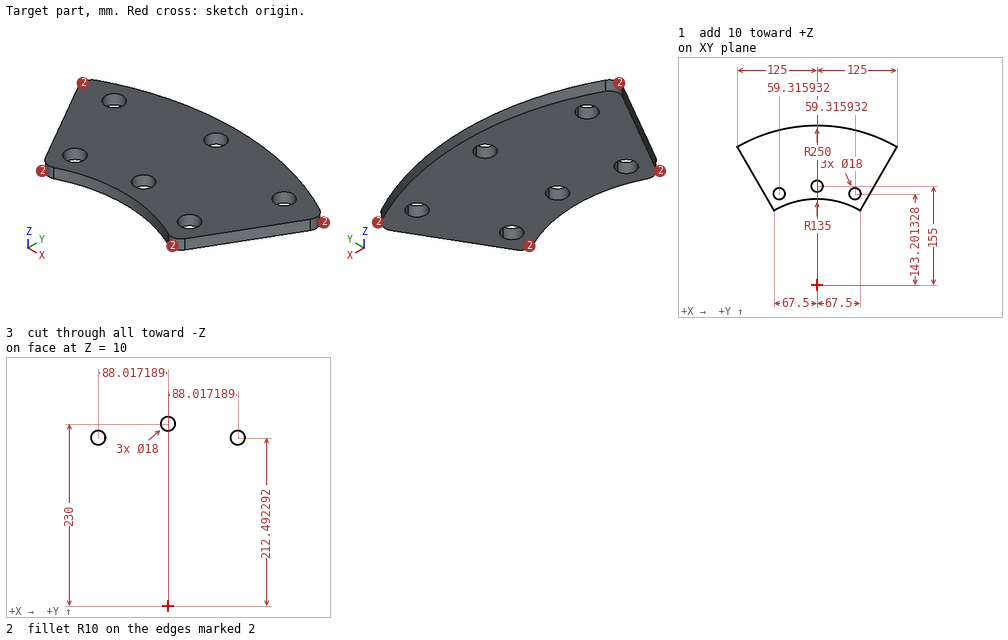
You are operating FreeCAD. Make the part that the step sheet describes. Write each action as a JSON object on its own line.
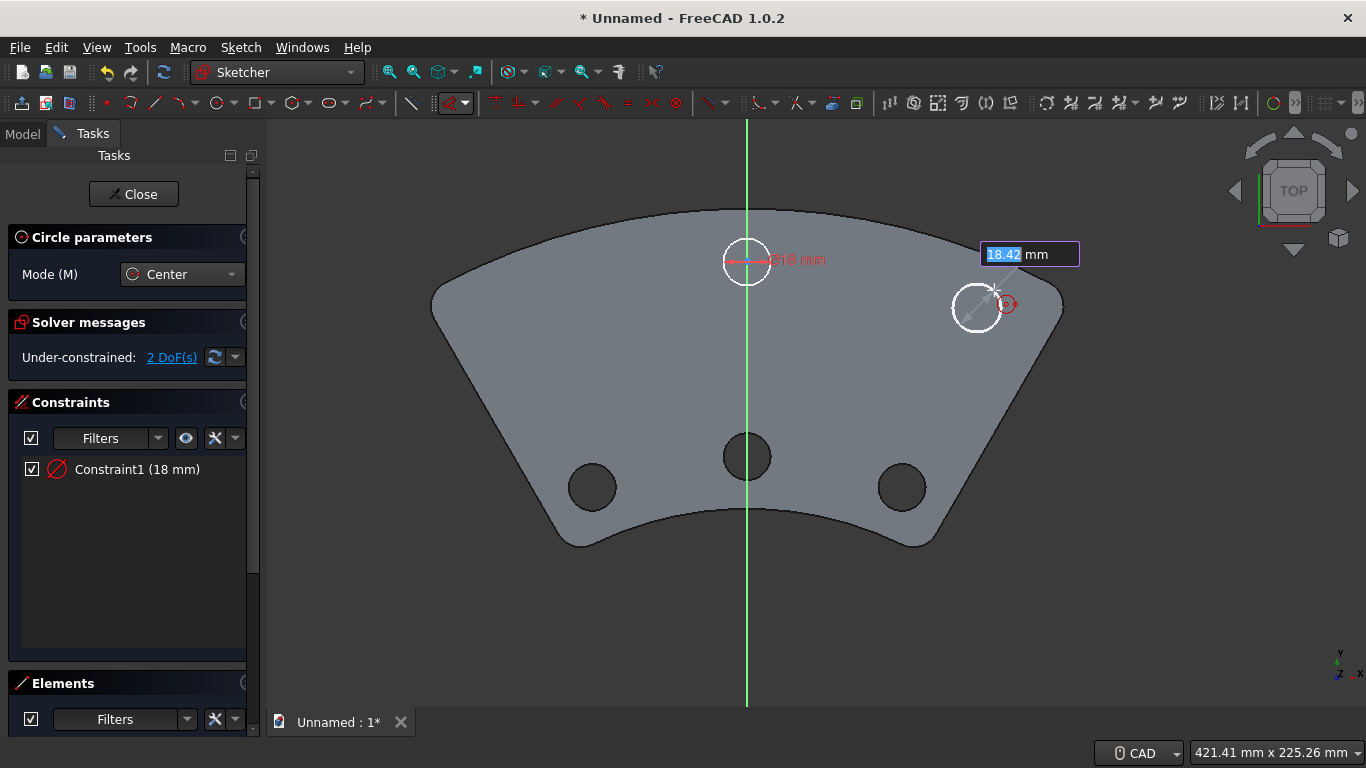
{"action": "type", "text": "18"}
{"action": "key", "text": "Return"}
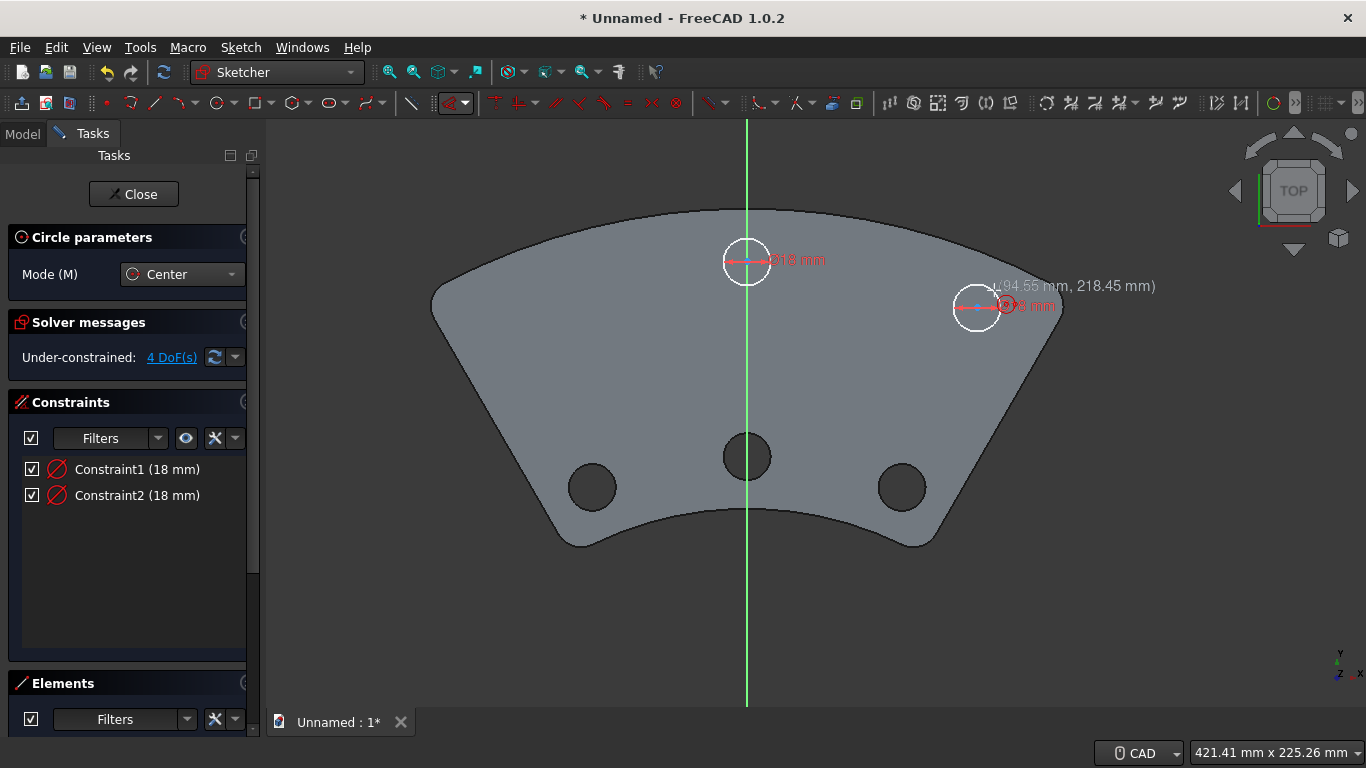
{"action": "left_click", "coordinate": [517, 307]}
{"action": "mouse_move", "coordinate": [534, 290]}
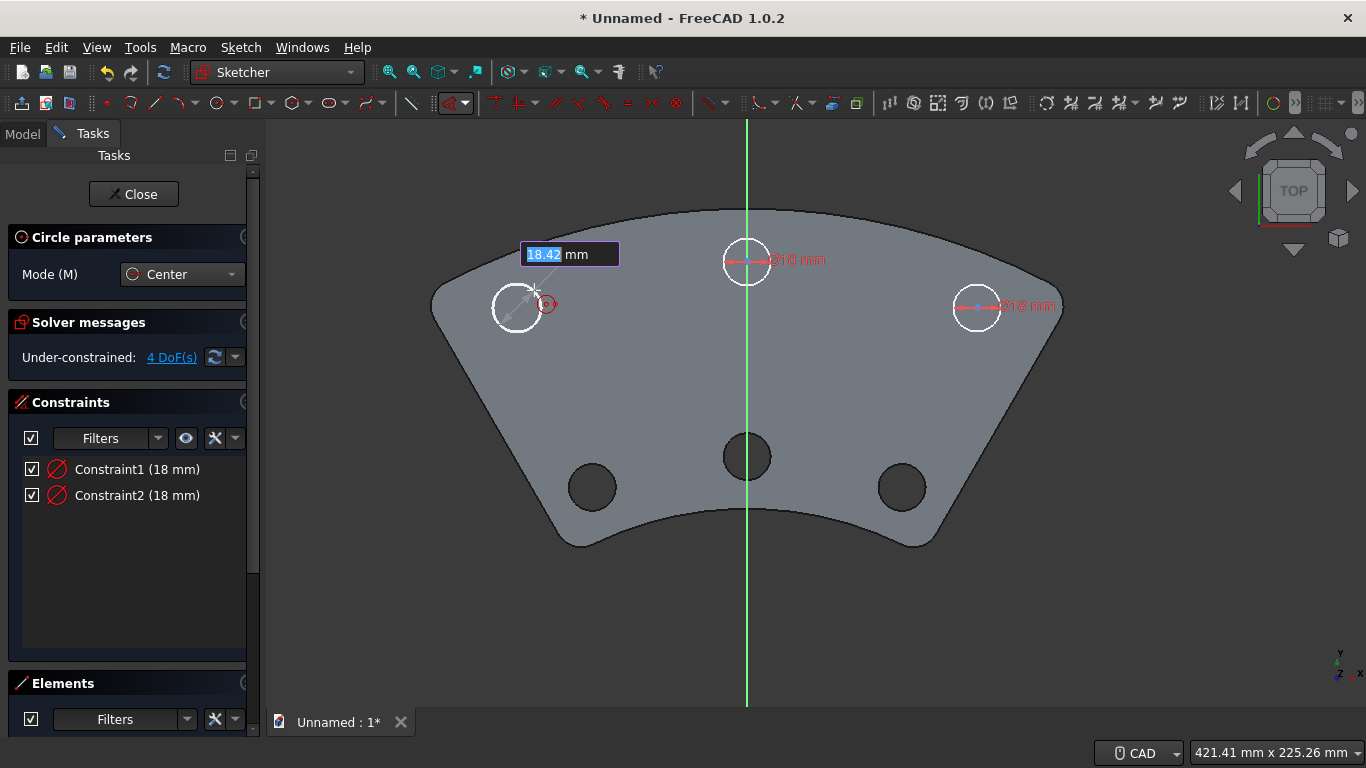
{"action": "type", "text": "18"}
{"action": "key", "text": "Return"}
{"action": "key", "text": "Escape"}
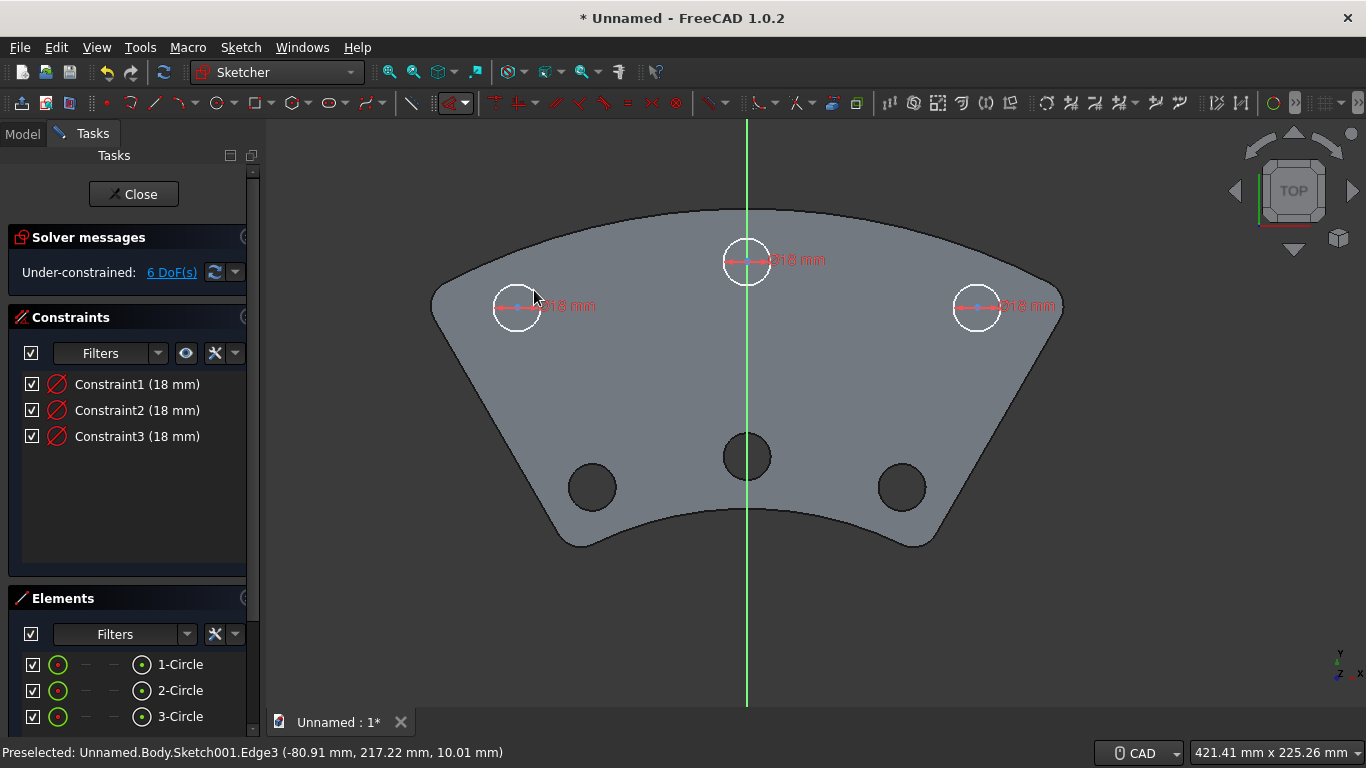
{"action": "left_click", "coordinate": [747, 262]}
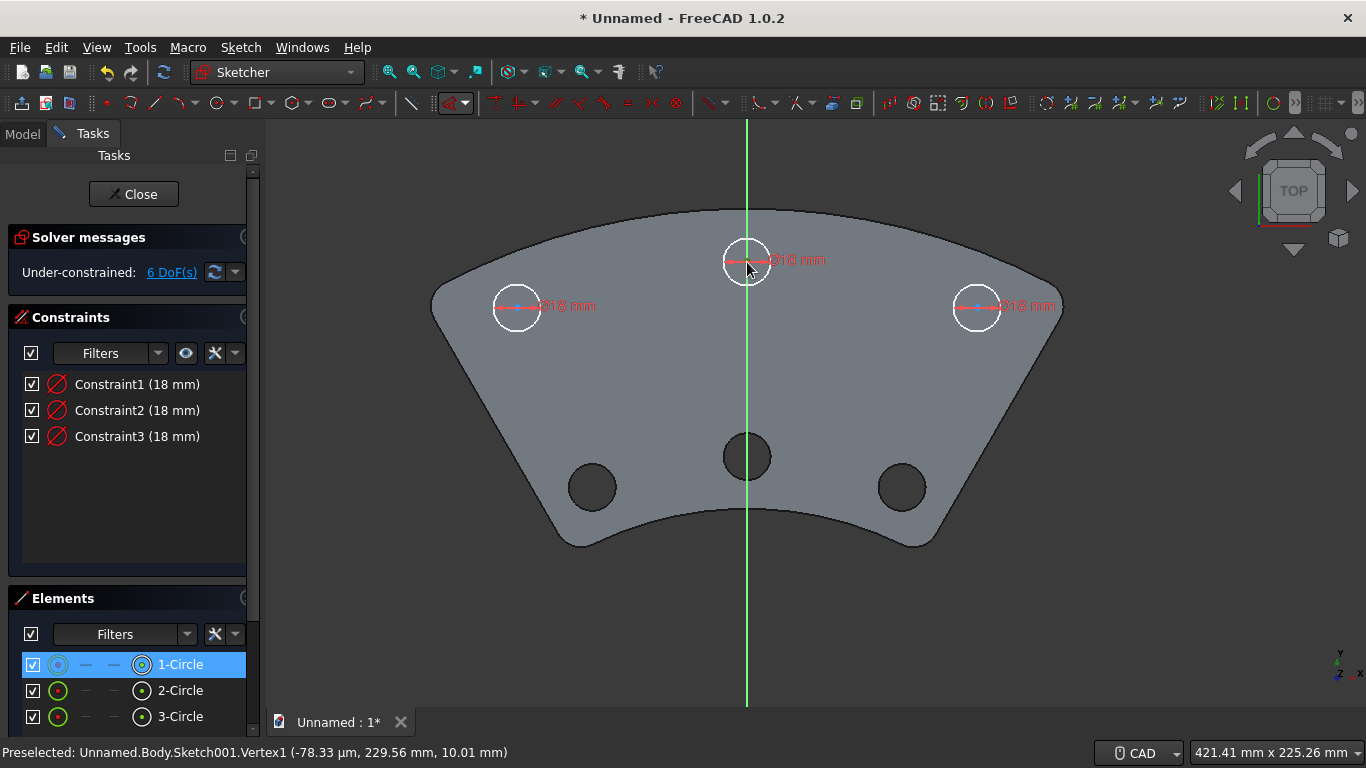
{"action": "left_click", "coordinate": [747, 641]}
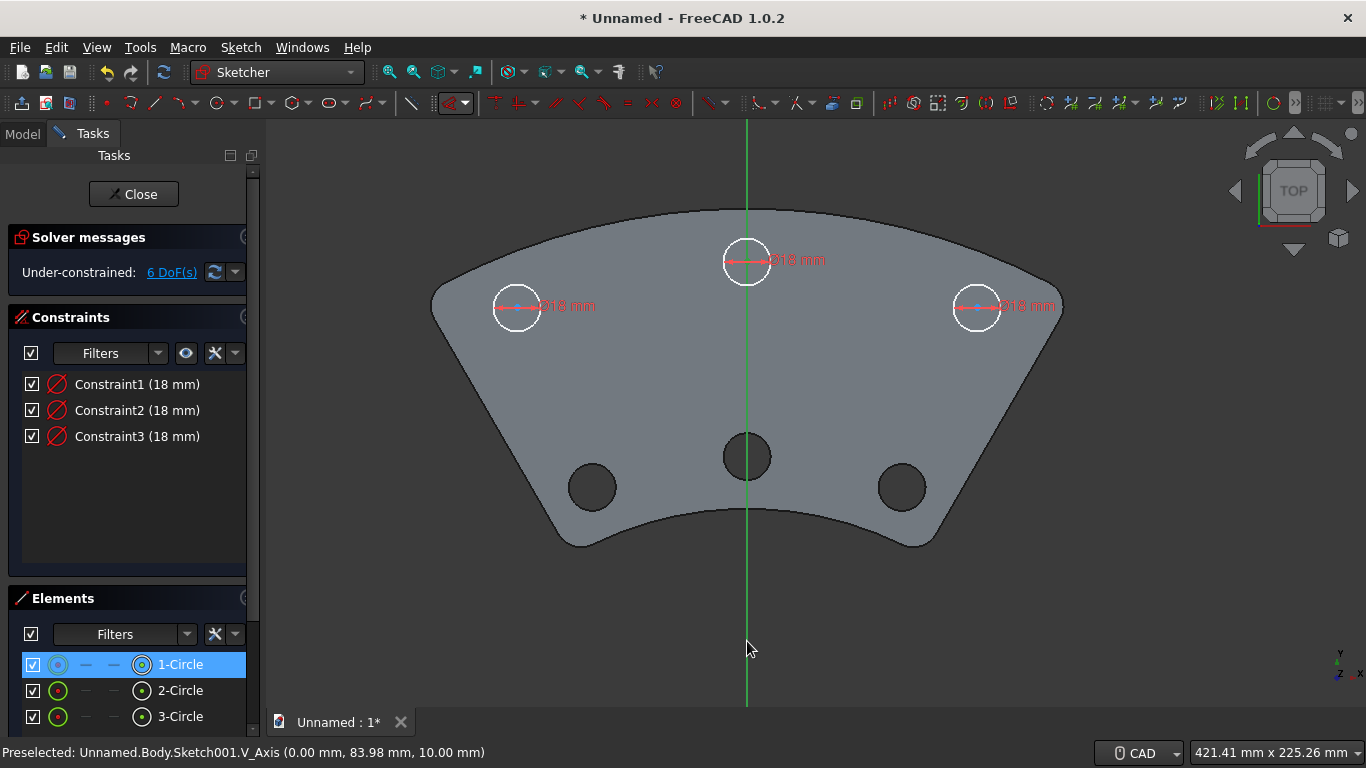
{"action": "left_click", "coordinate": [496, 104]}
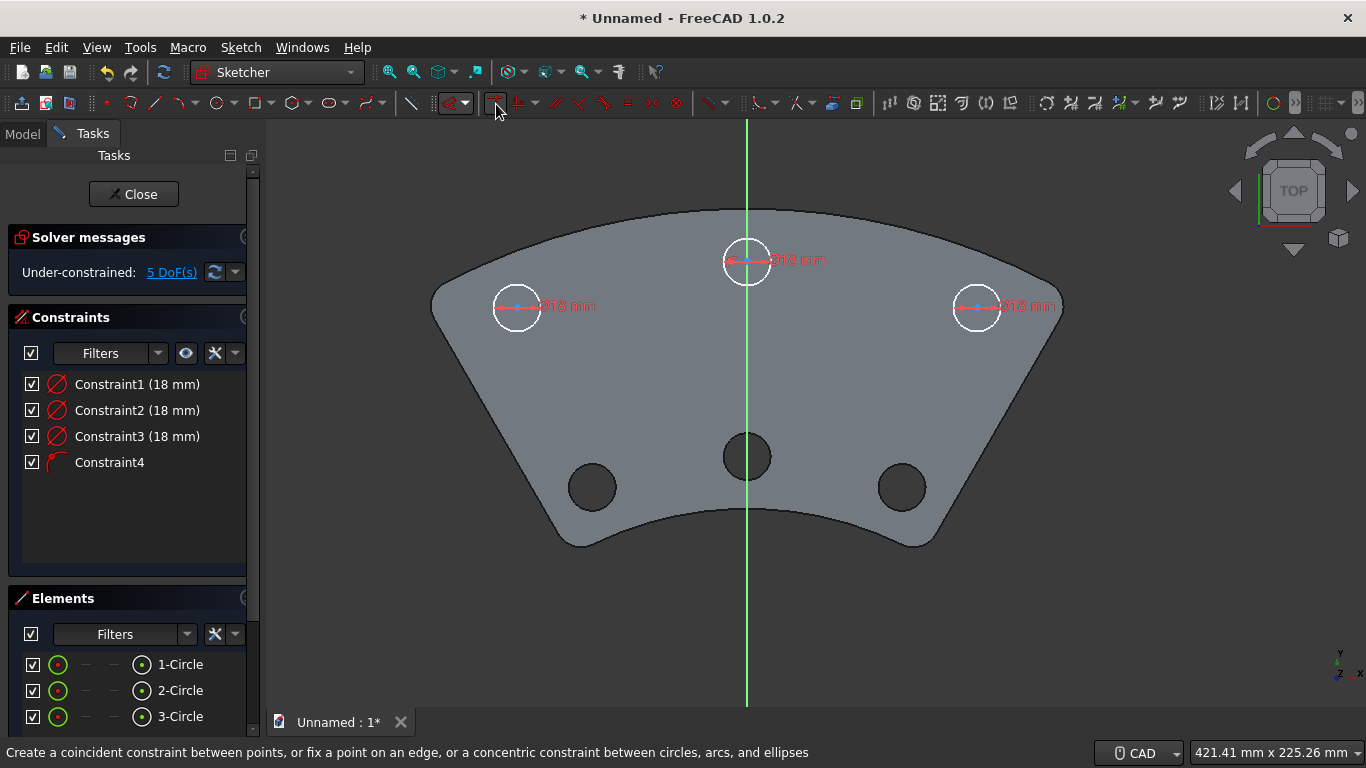
{"action": "left_click", "coordinate": [977, 308]}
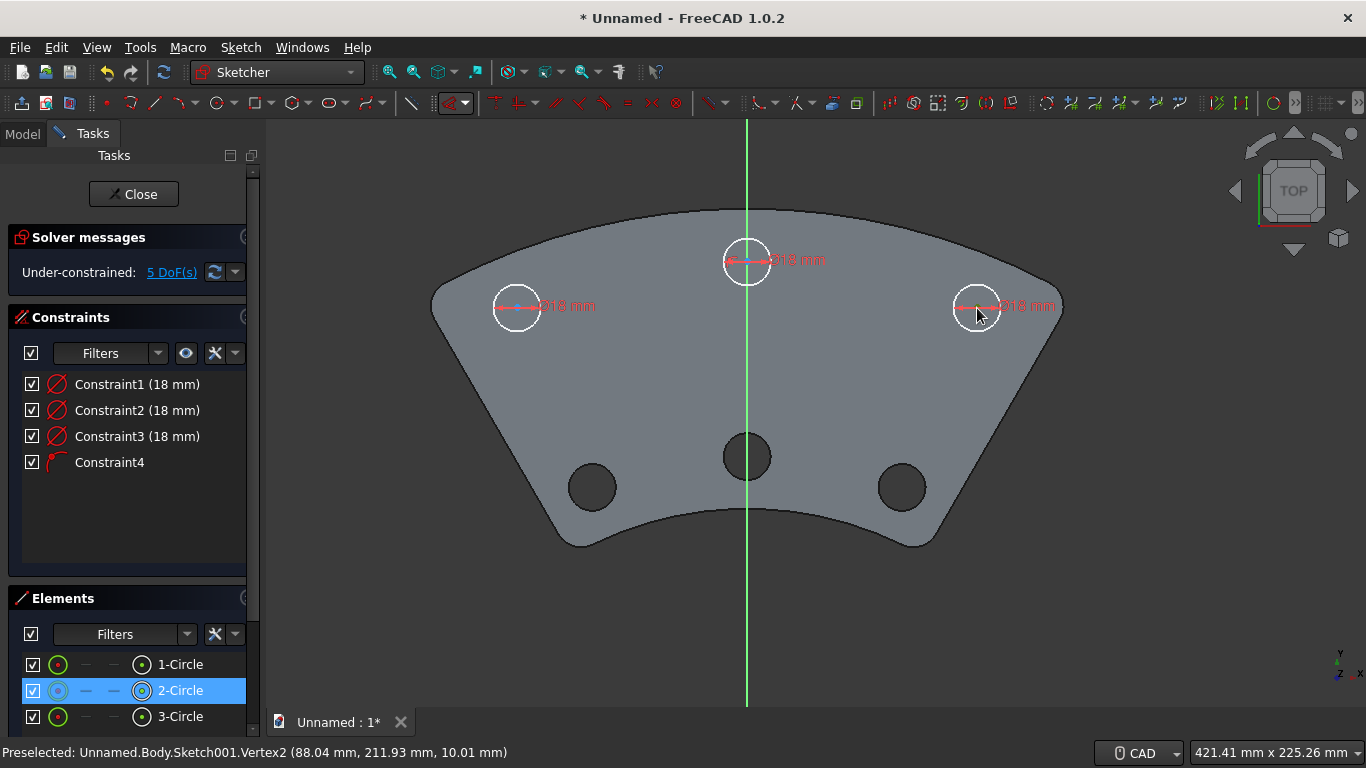
{"action": "left_click", "coordinate": [517, 308]}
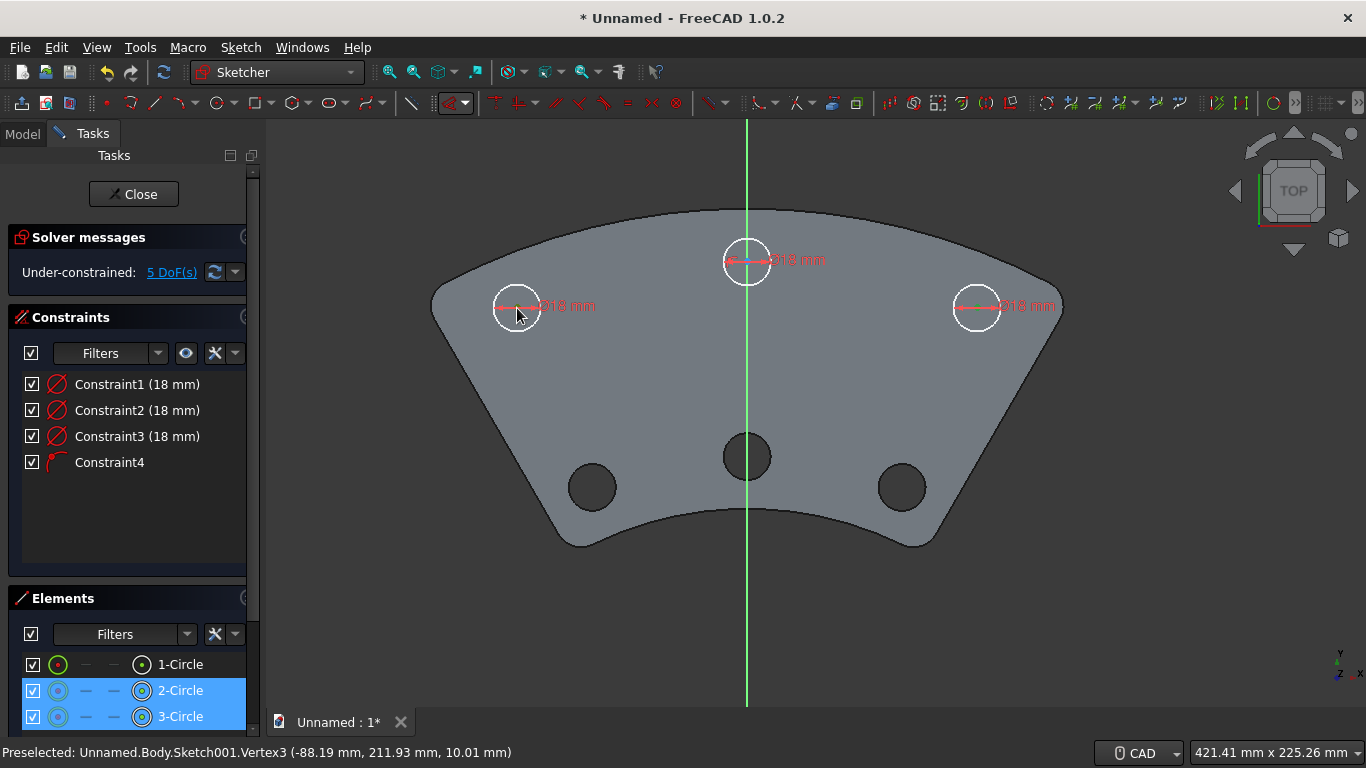
{"action": "left_click", "coordinate": [538, 104]}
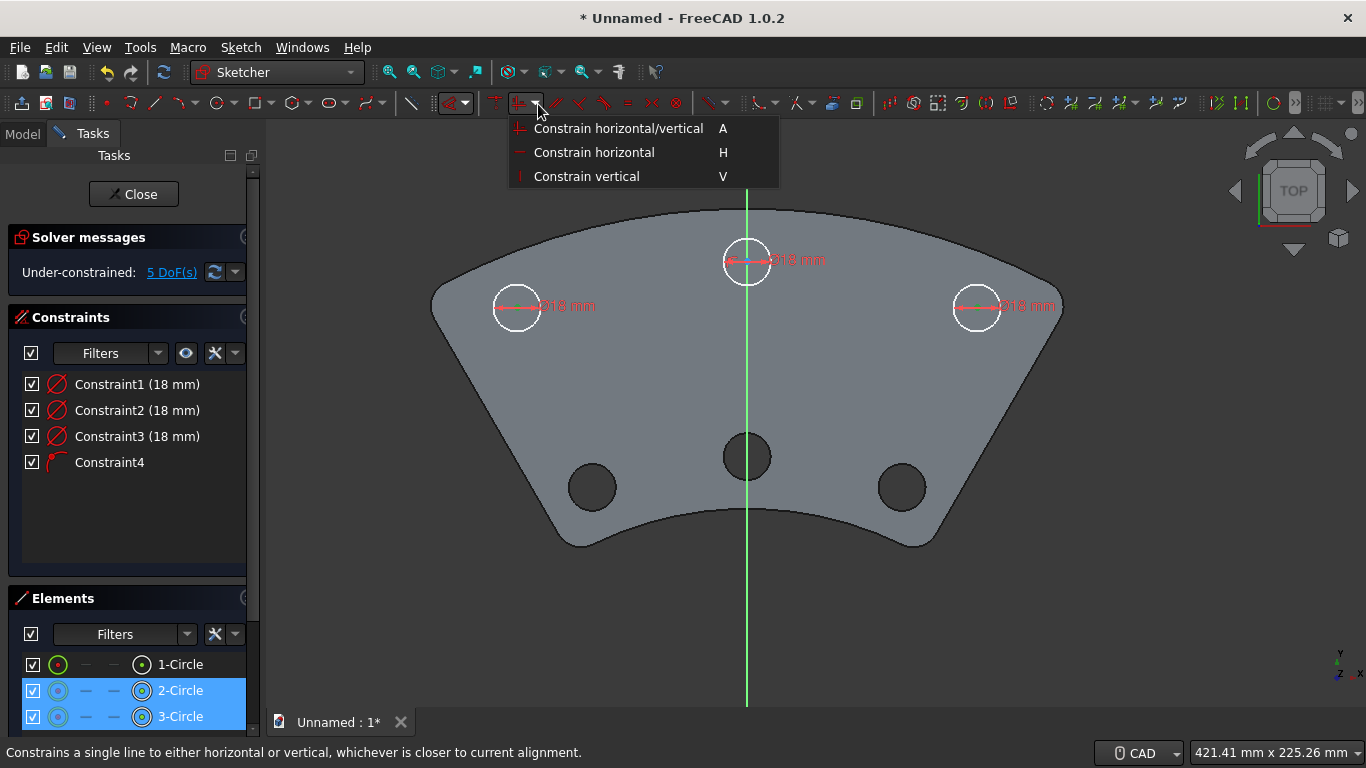
{"action": "left_click", "coordinate": [644, 152]}